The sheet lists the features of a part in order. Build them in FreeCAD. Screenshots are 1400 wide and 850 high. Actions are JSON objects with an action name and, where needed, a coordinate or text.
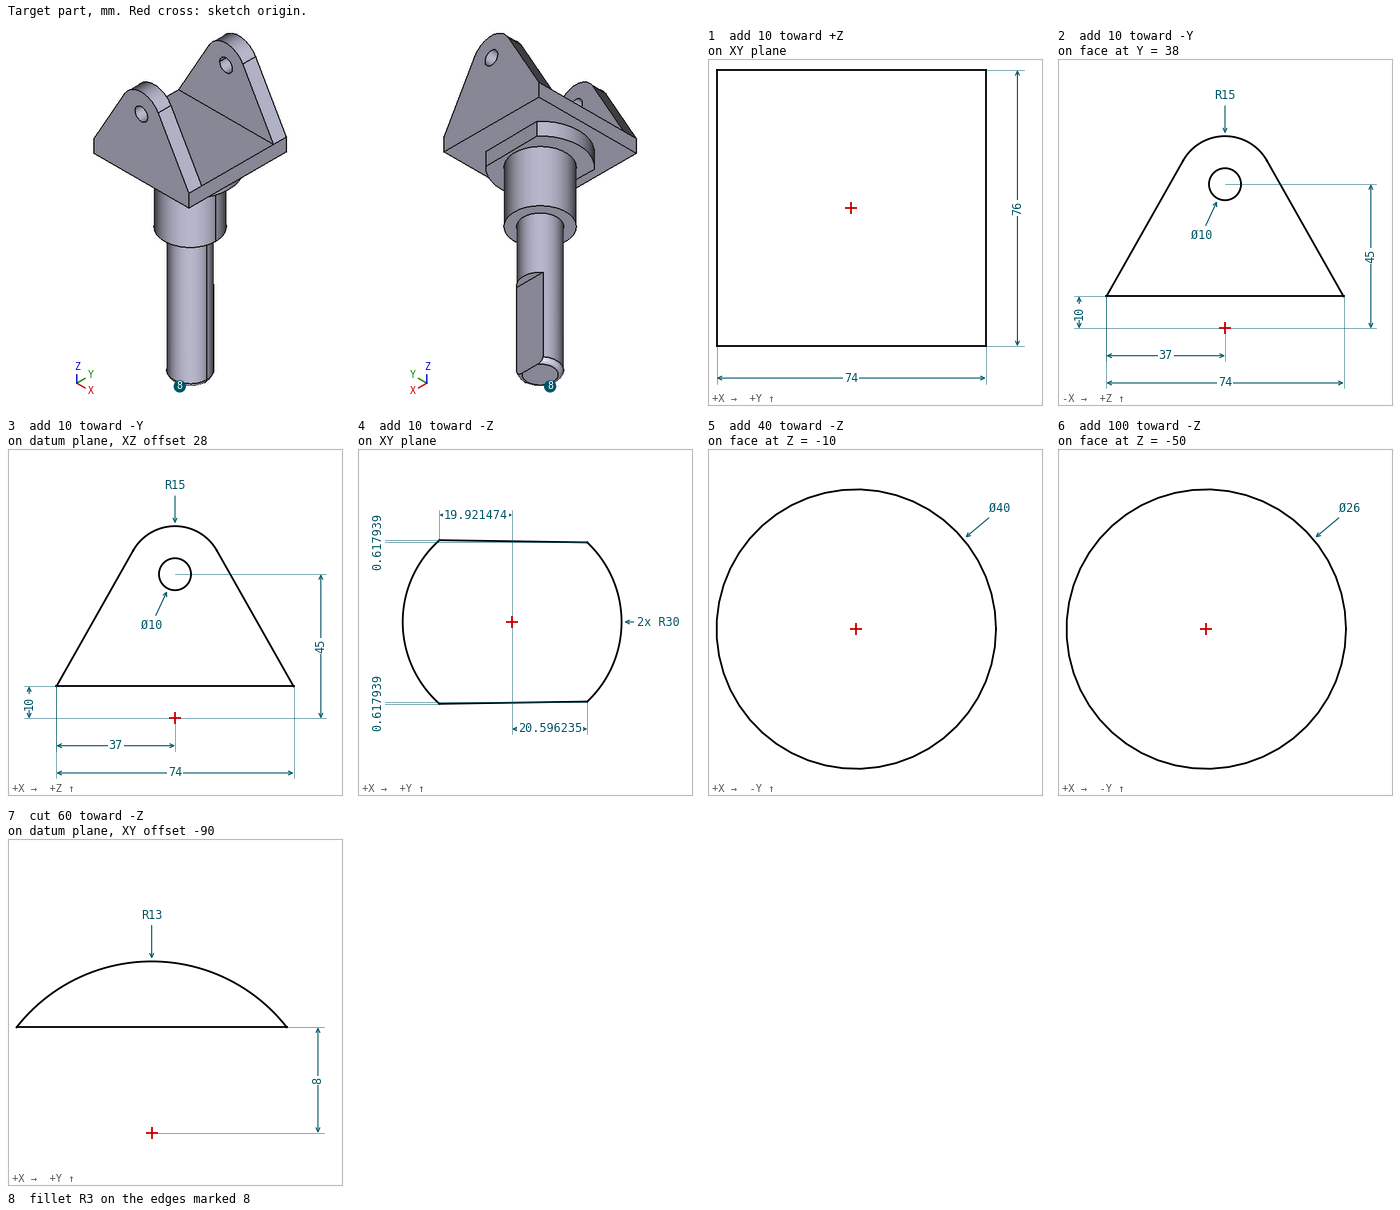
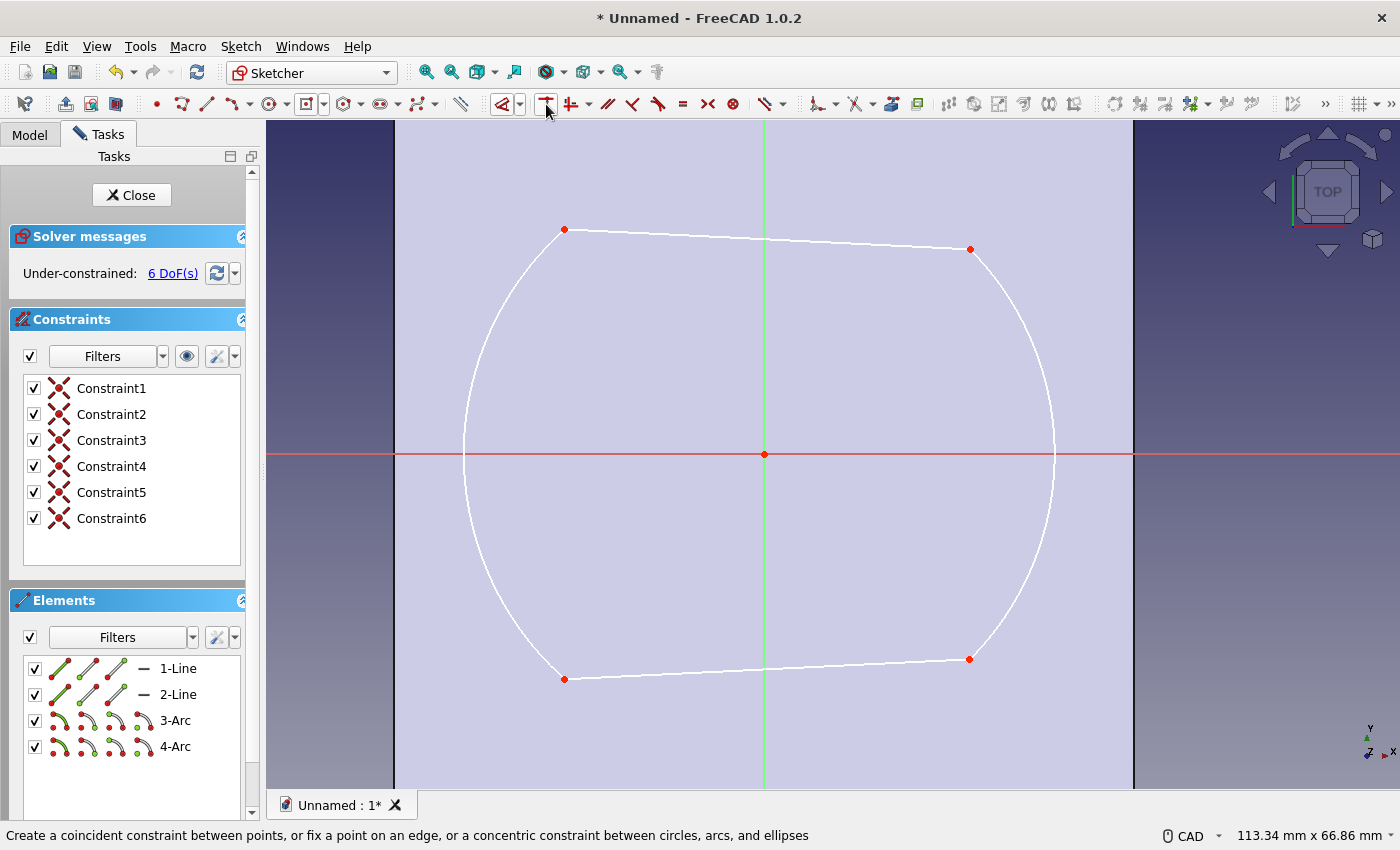
{"action": "left_click", "coordinate": [1041, 544]}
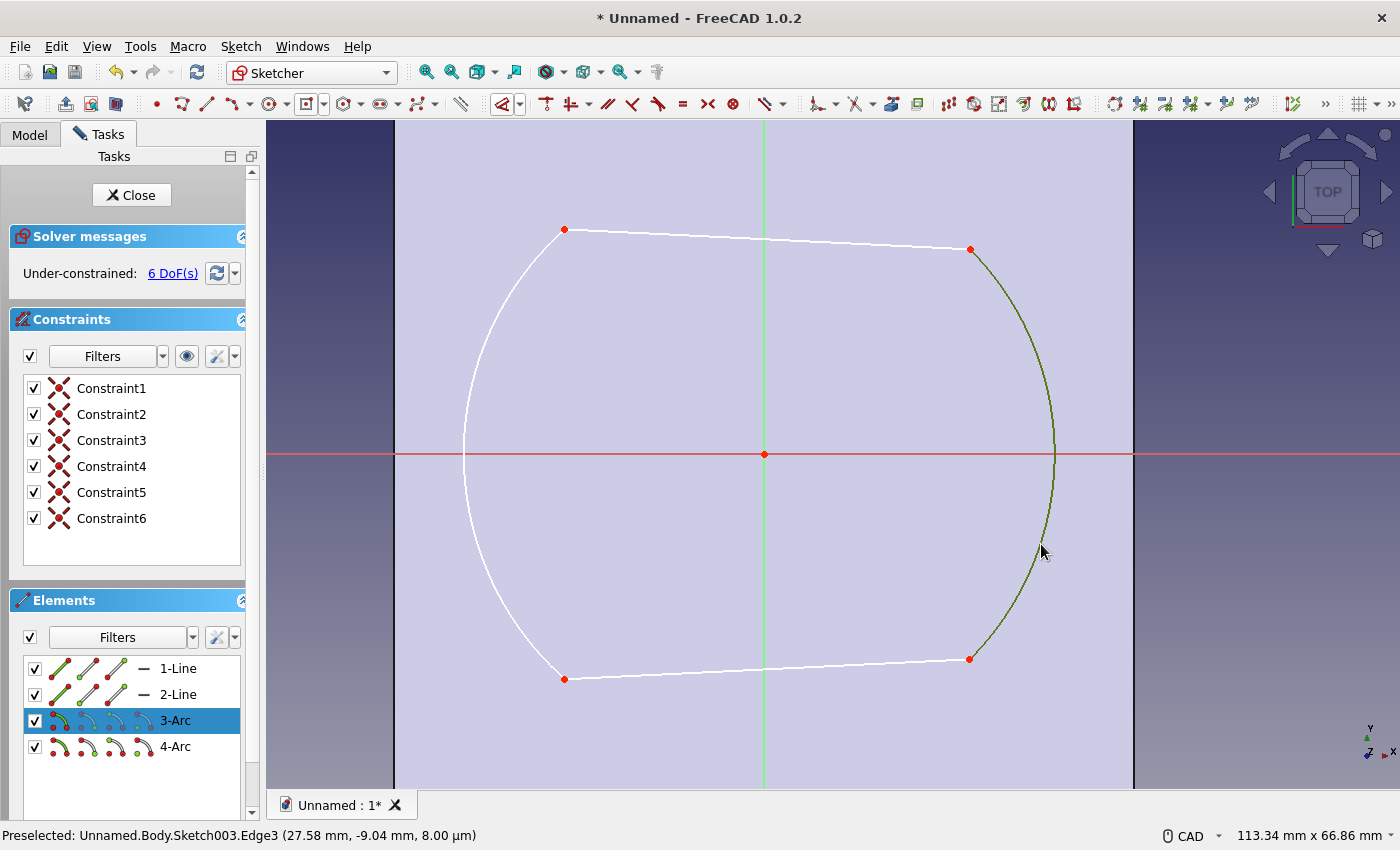
{"action": "left_click", "coordinate": [481, 355]}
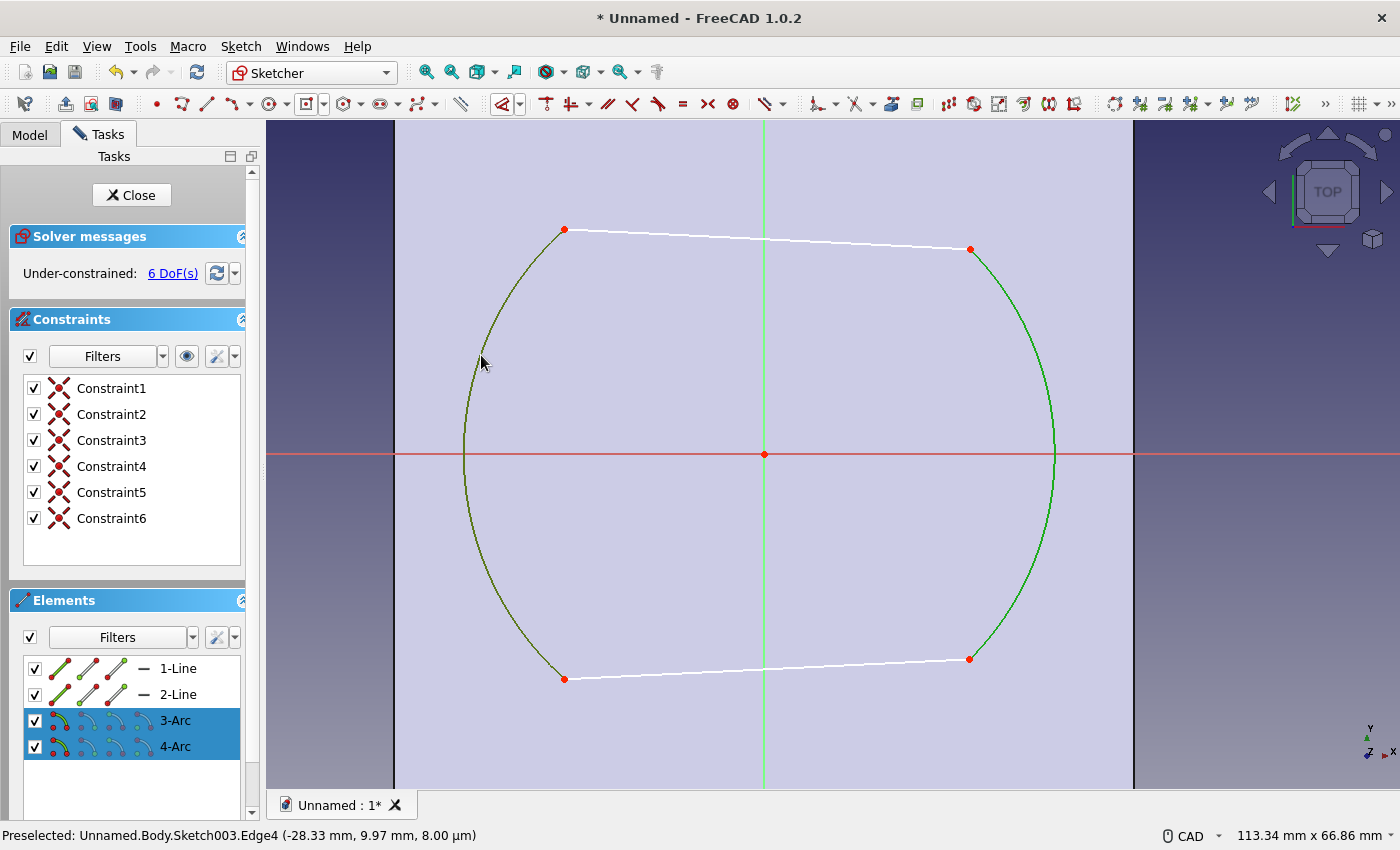
{"action": "left_click", "coordinate": [683, 104]}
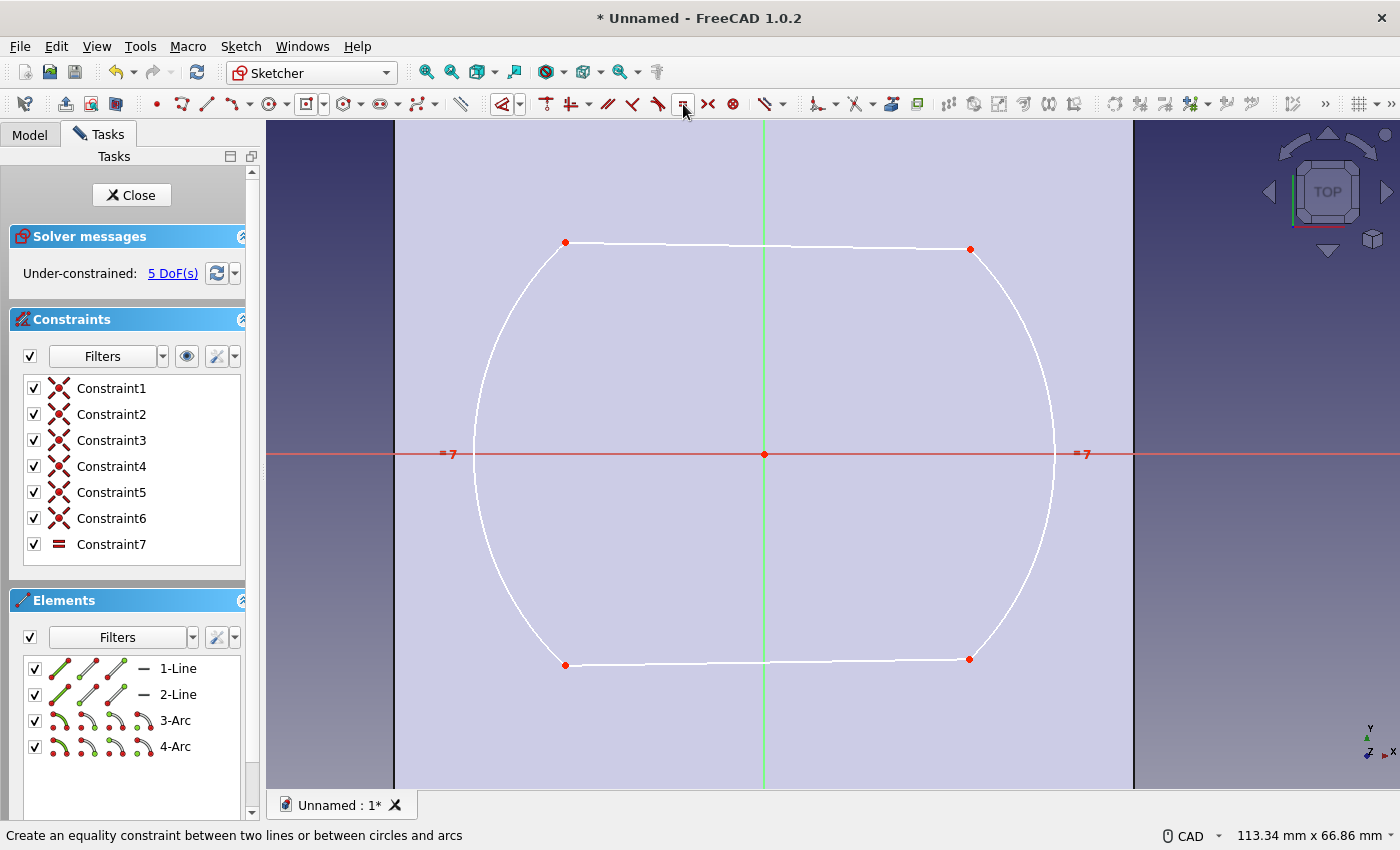
{"action": "left_click", "coordinate": [1041, 544]}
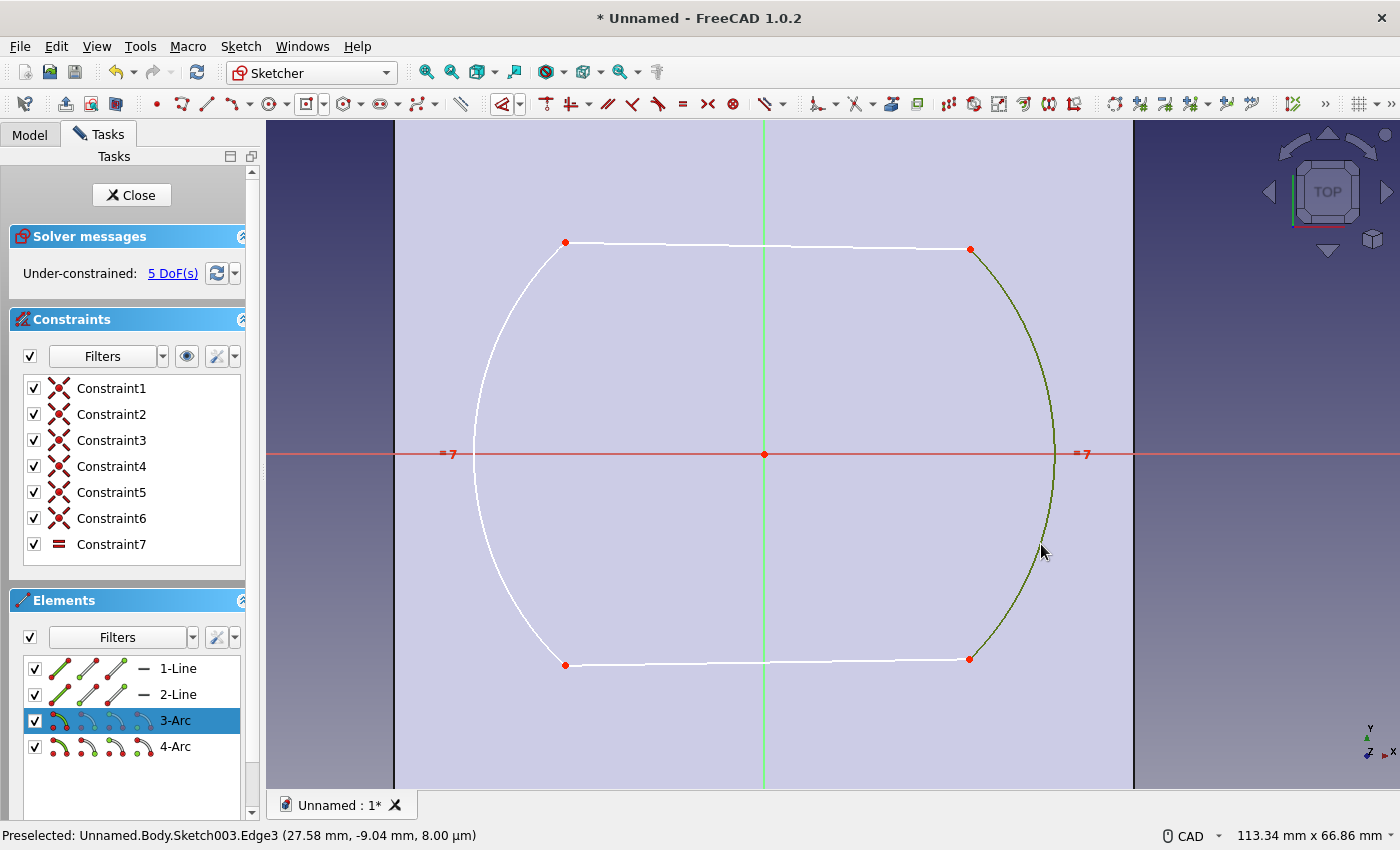
{"action": "left_click", "coordinate": [520, 104]}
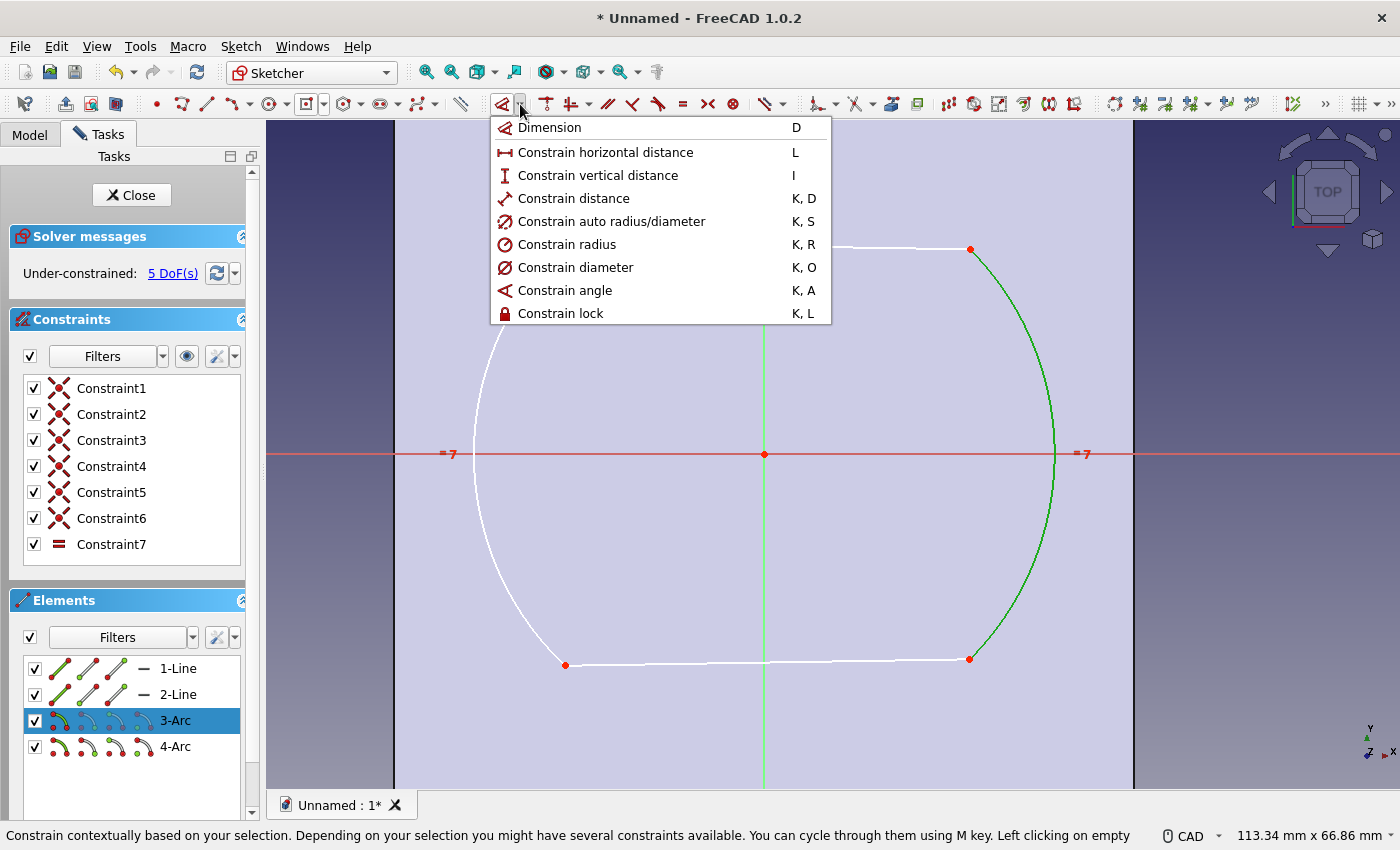
{"action": "left_click", "coordinate": [661, 244]}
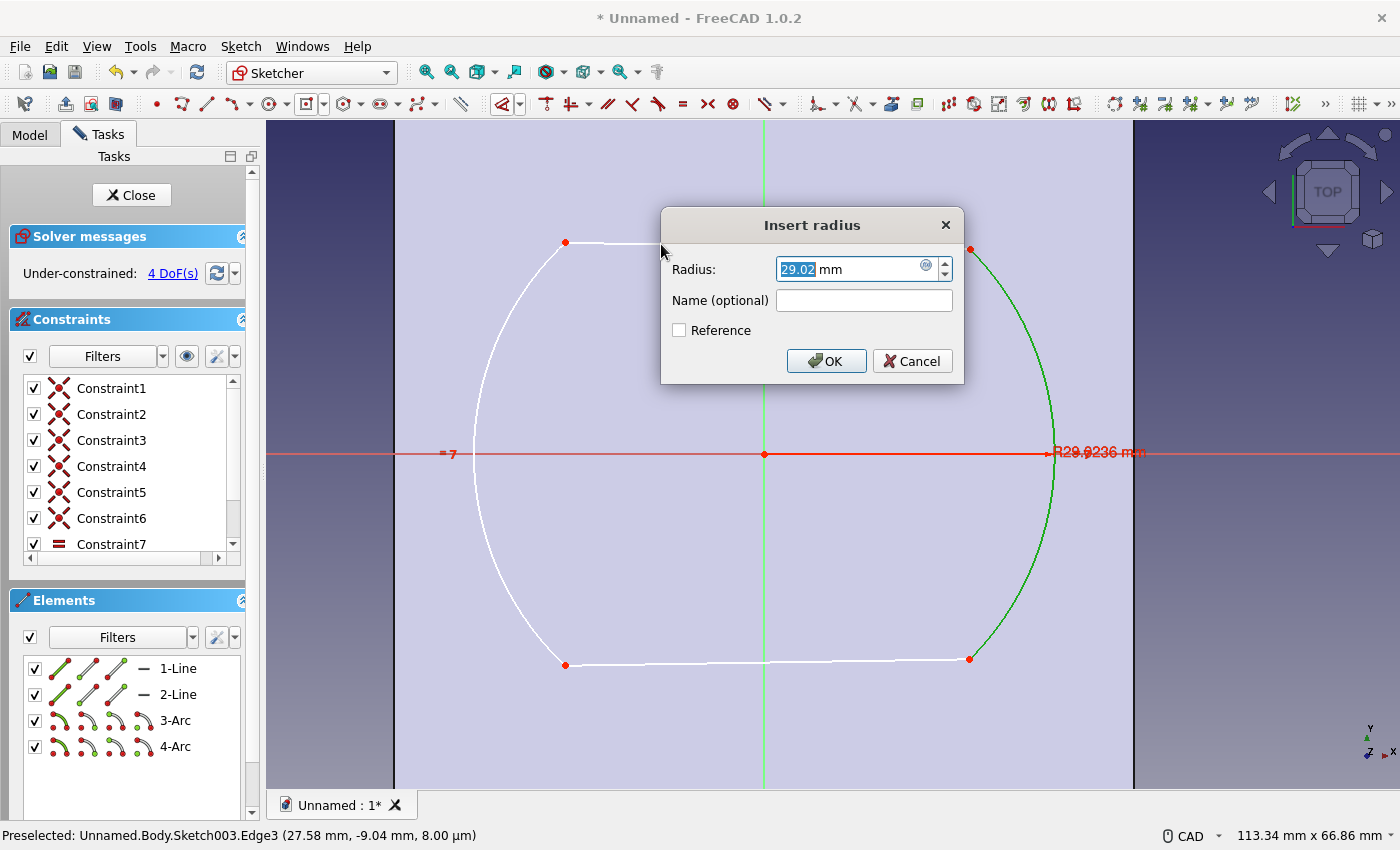
{"action": "type", "text": "30"}
{"action": "key", "text": "Return"}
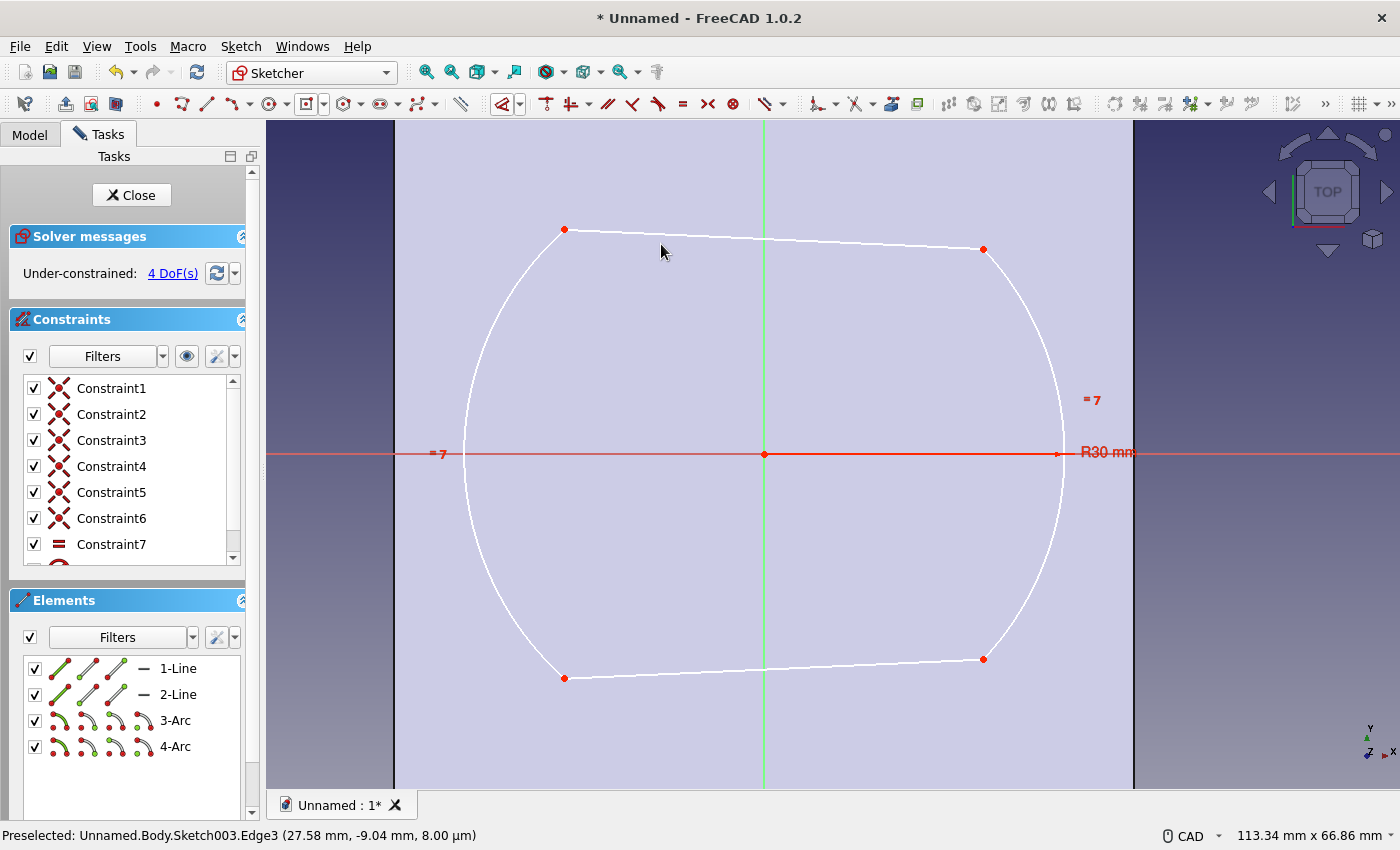
{"action": "scroll", "coordinate": [690, 236], "scroll_direction": "up", "scroll_amount": 10}